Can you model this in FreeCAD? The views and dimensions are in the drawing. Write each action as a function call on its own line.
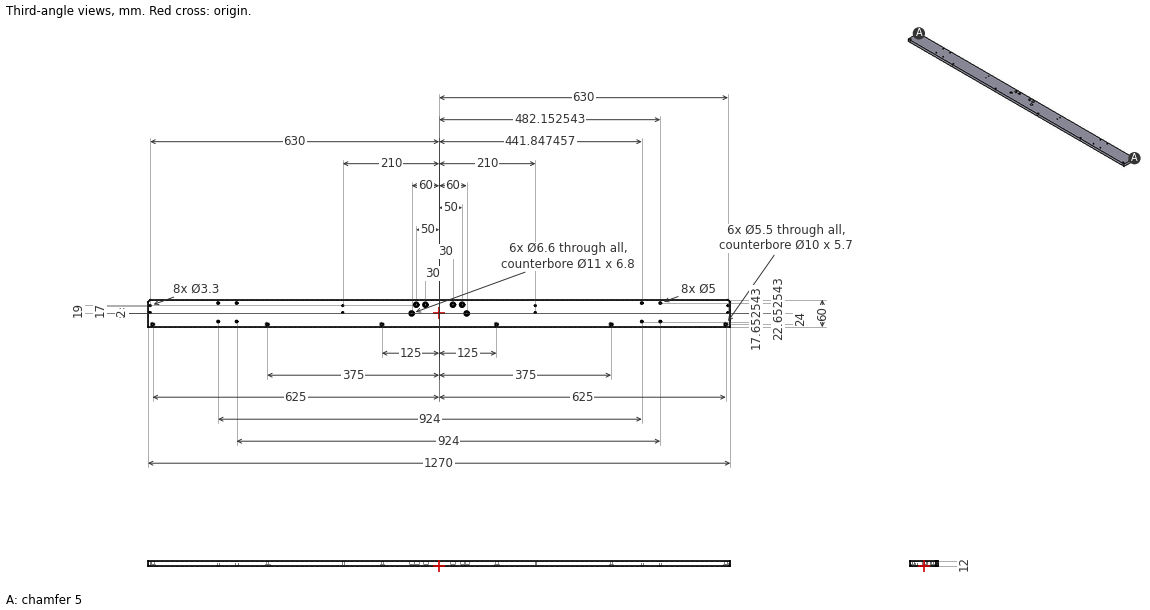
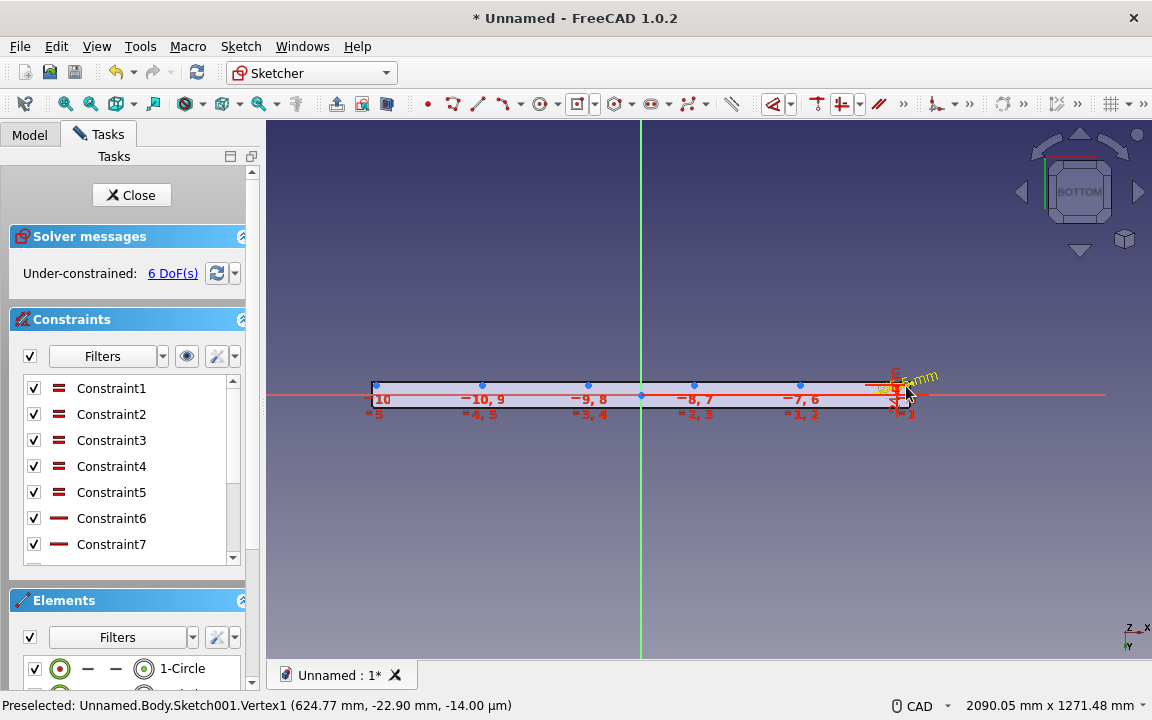
click(906, 385)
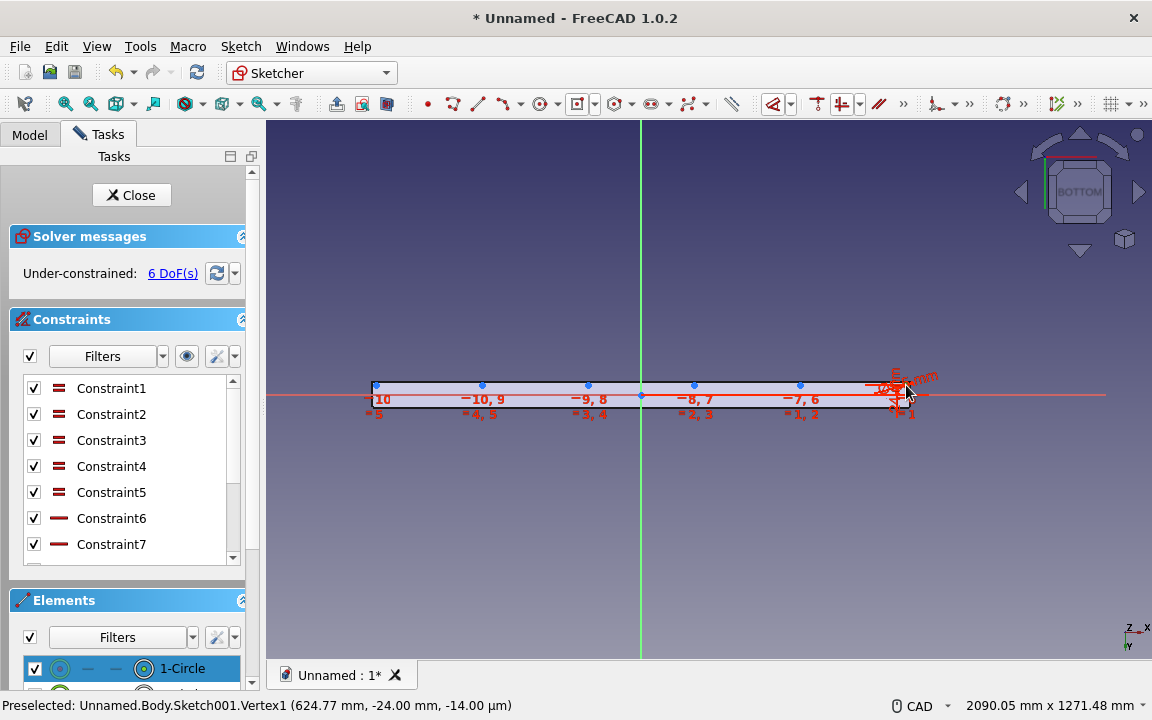
key(l)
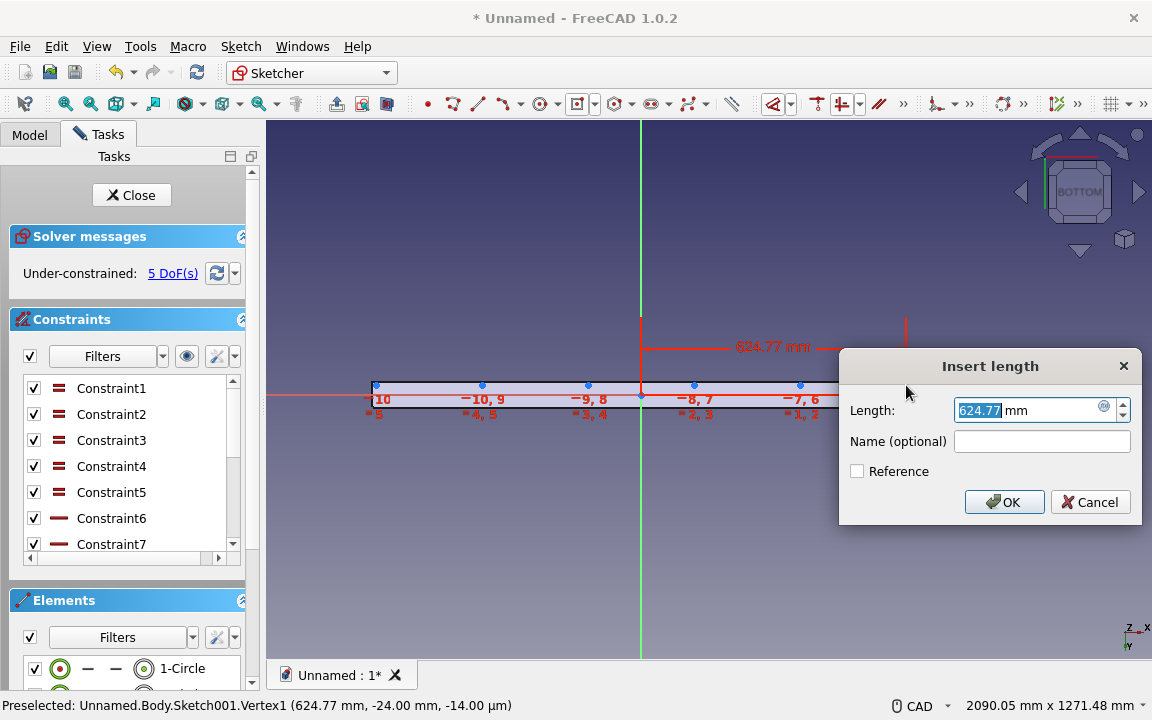
text(625)
key(Return)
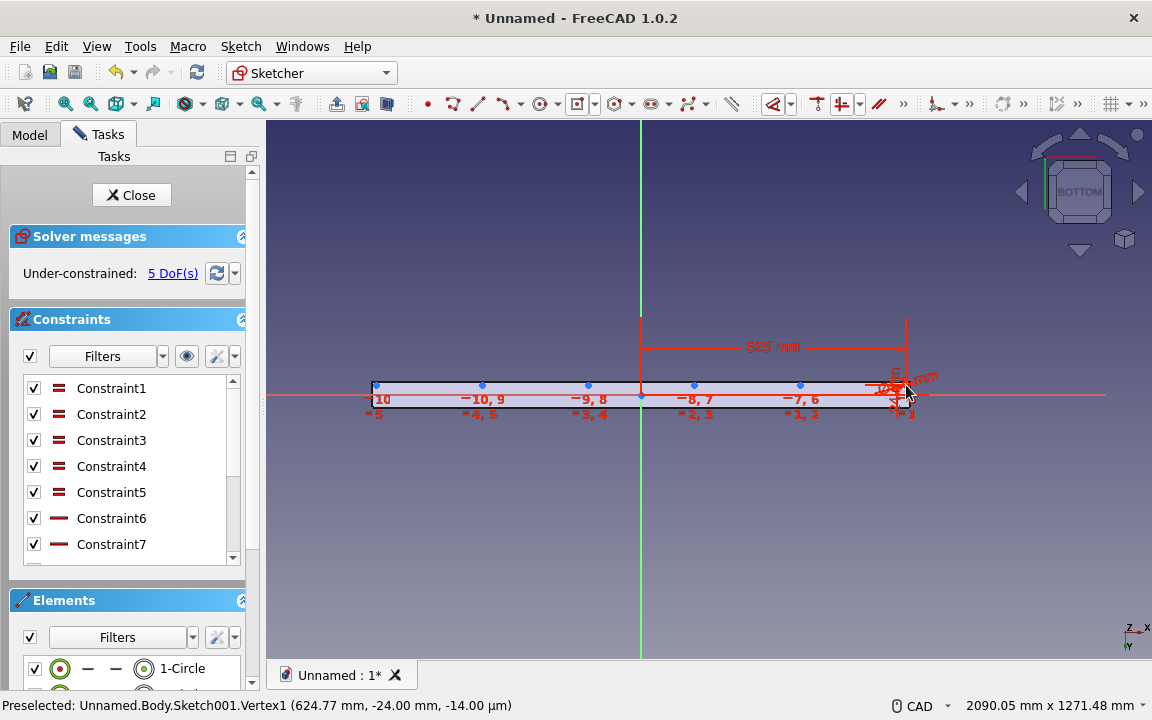
click(800, 385)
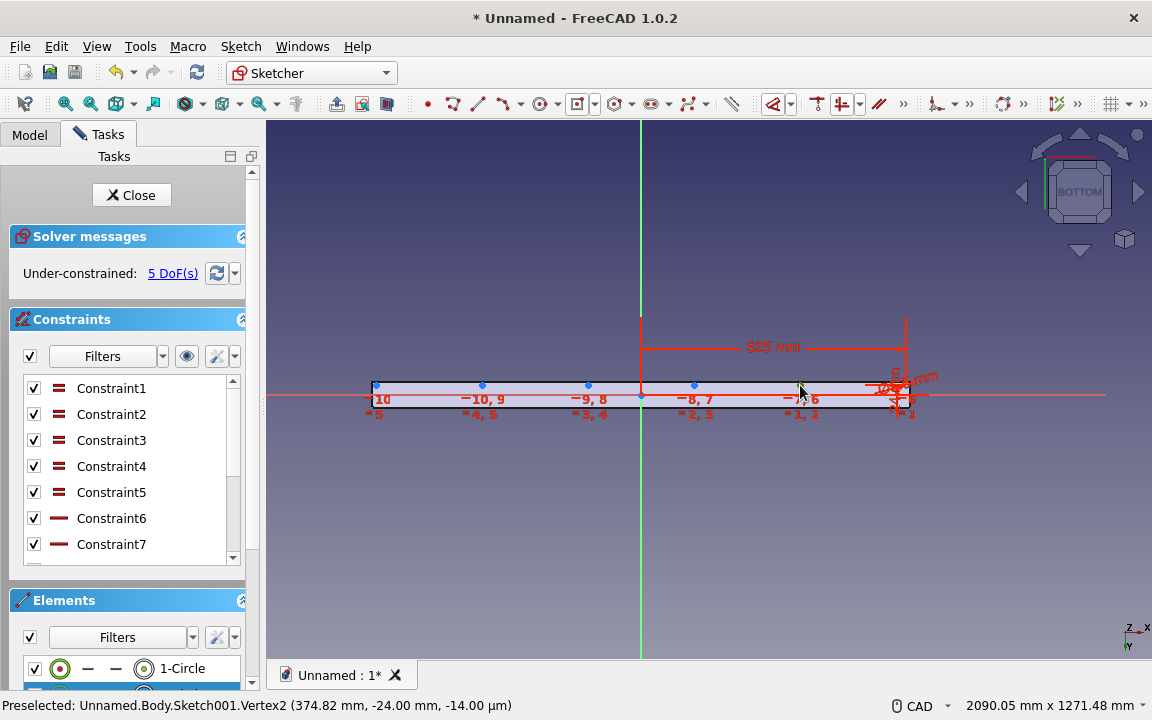
click(790, 104)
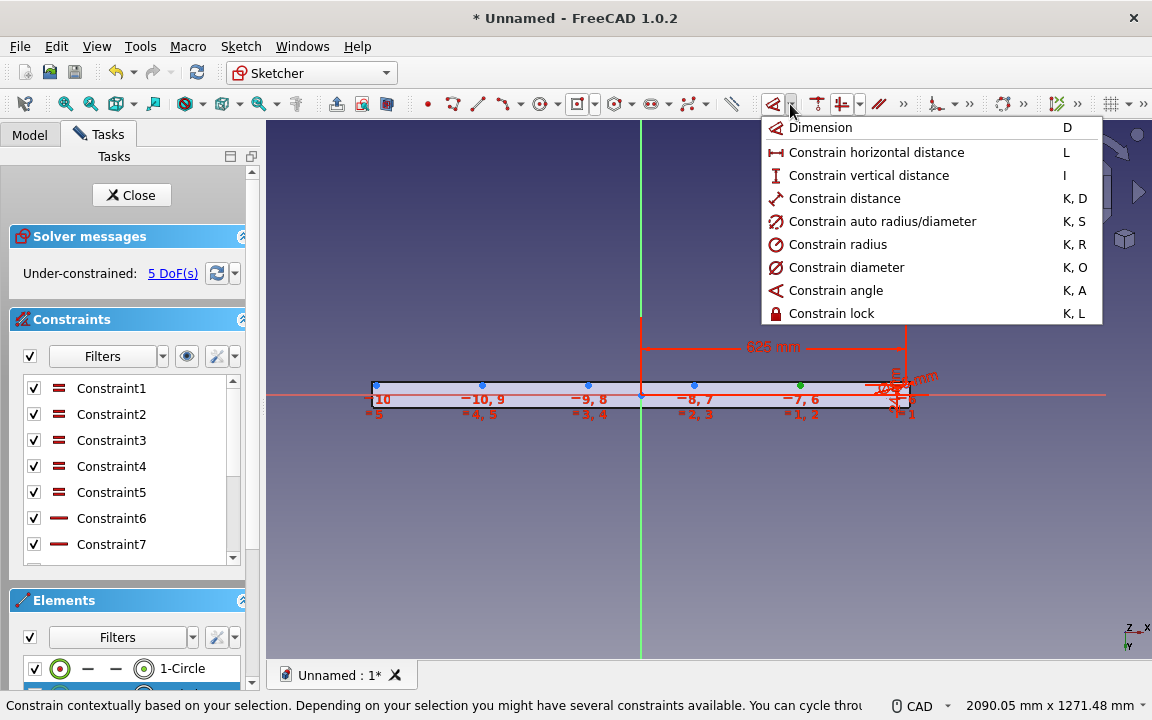
click(932, 152)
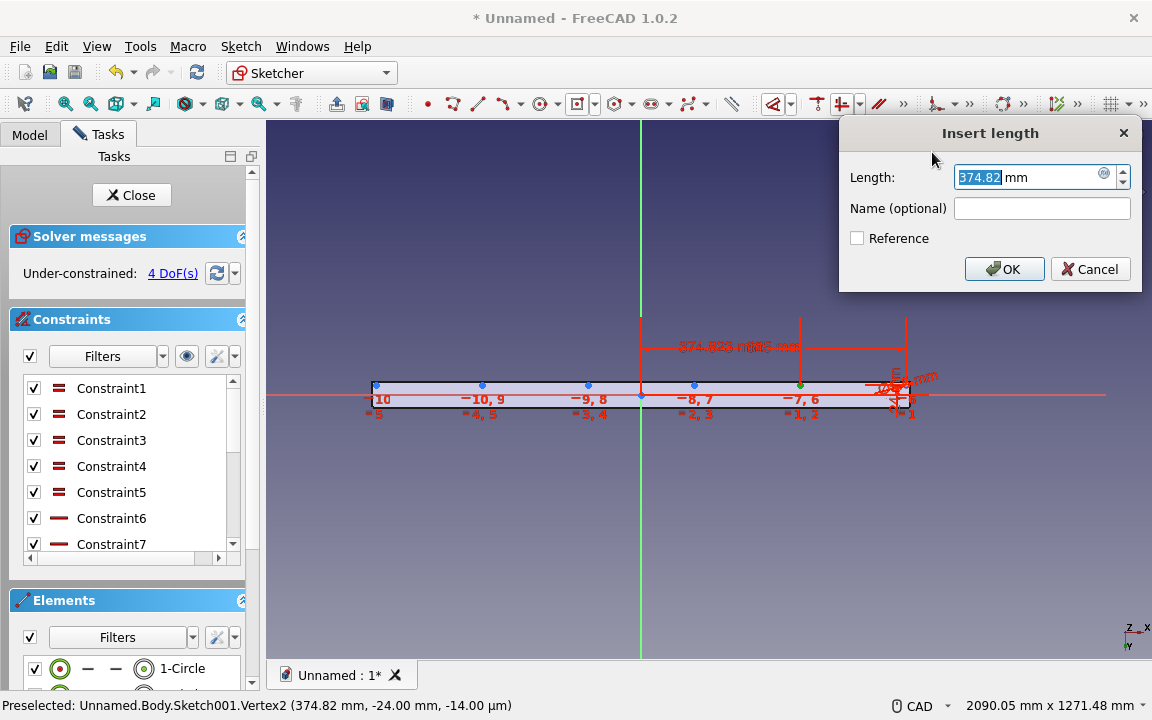
text(375)
key(Return)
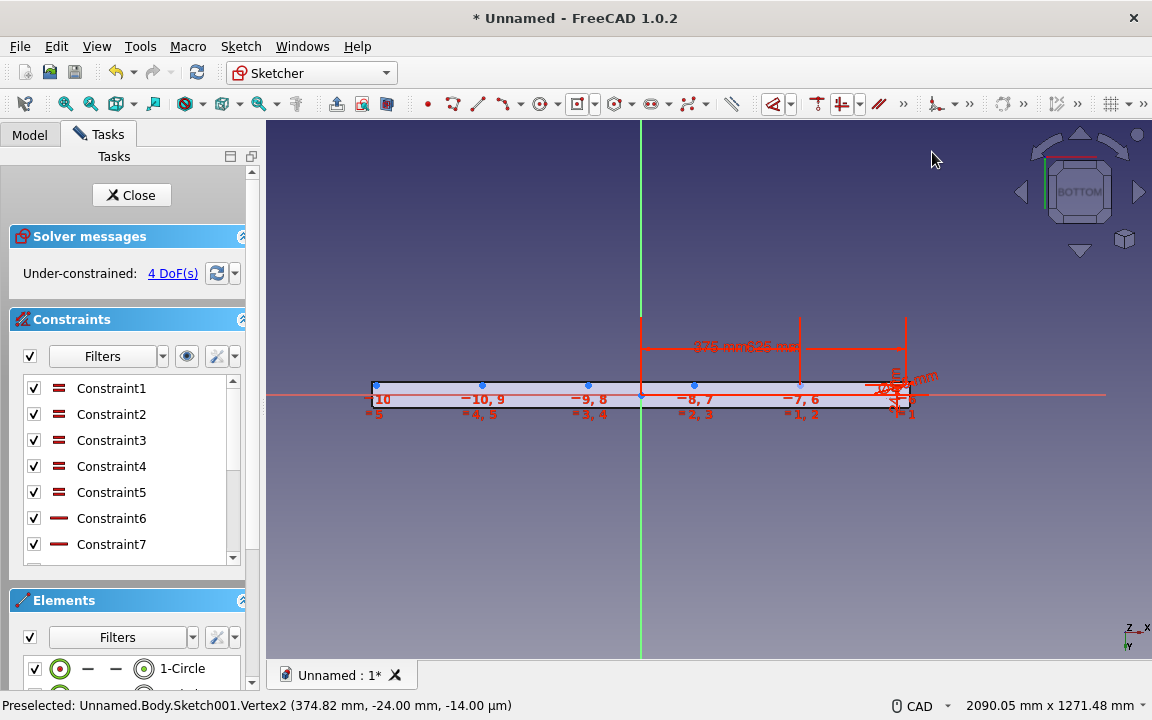
click(694, 385)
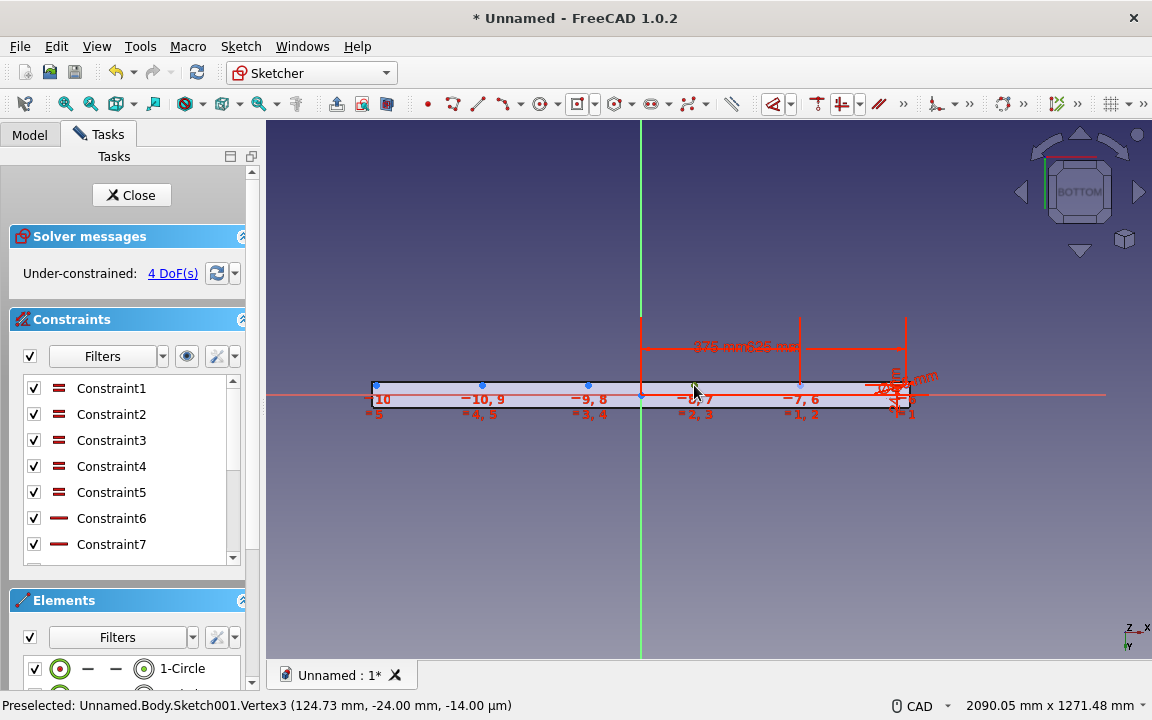
key(l)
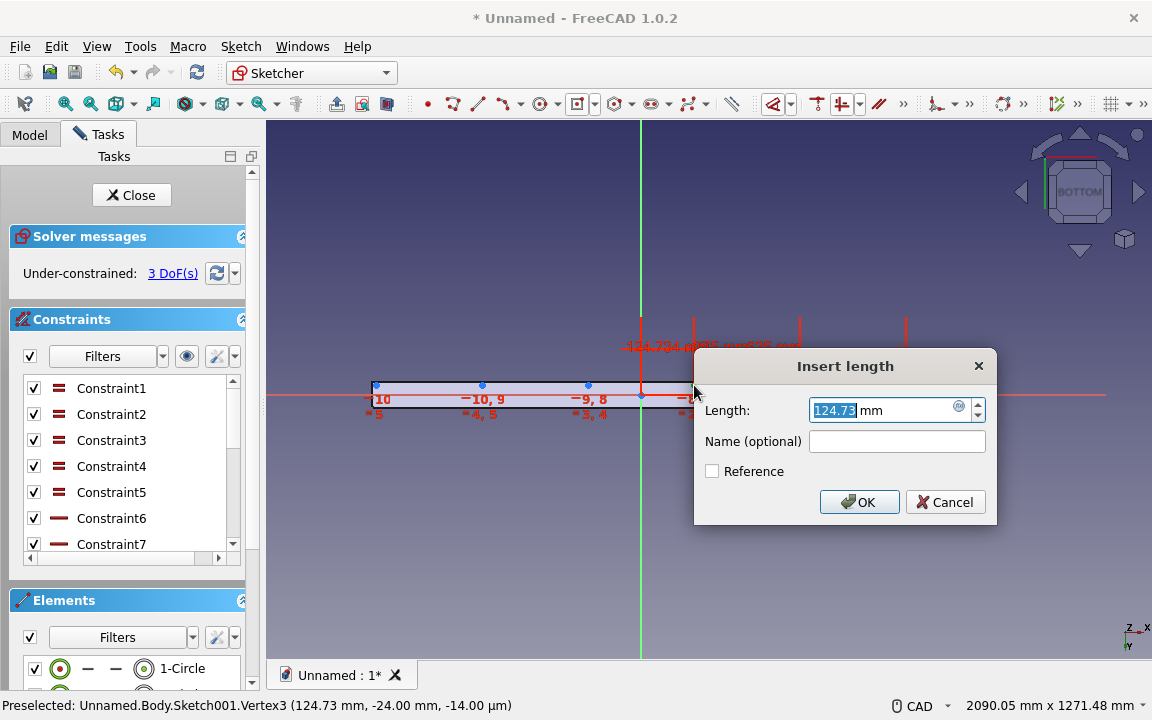
text(125)
key(Return)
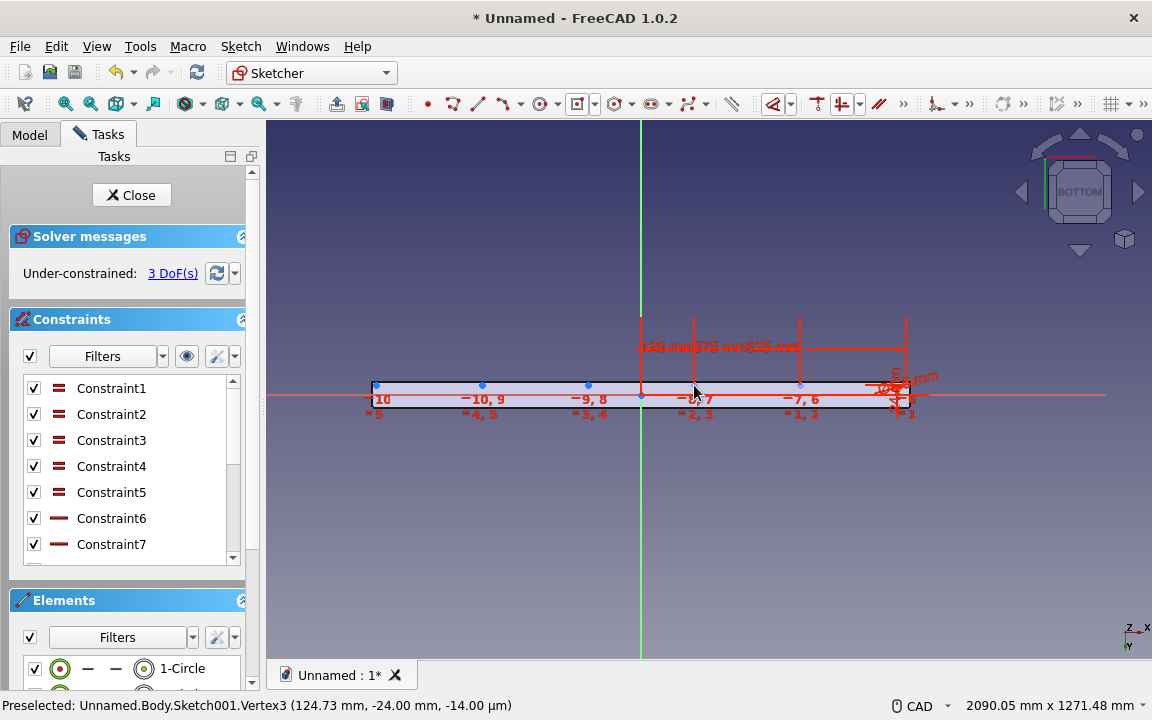
click(588, 385)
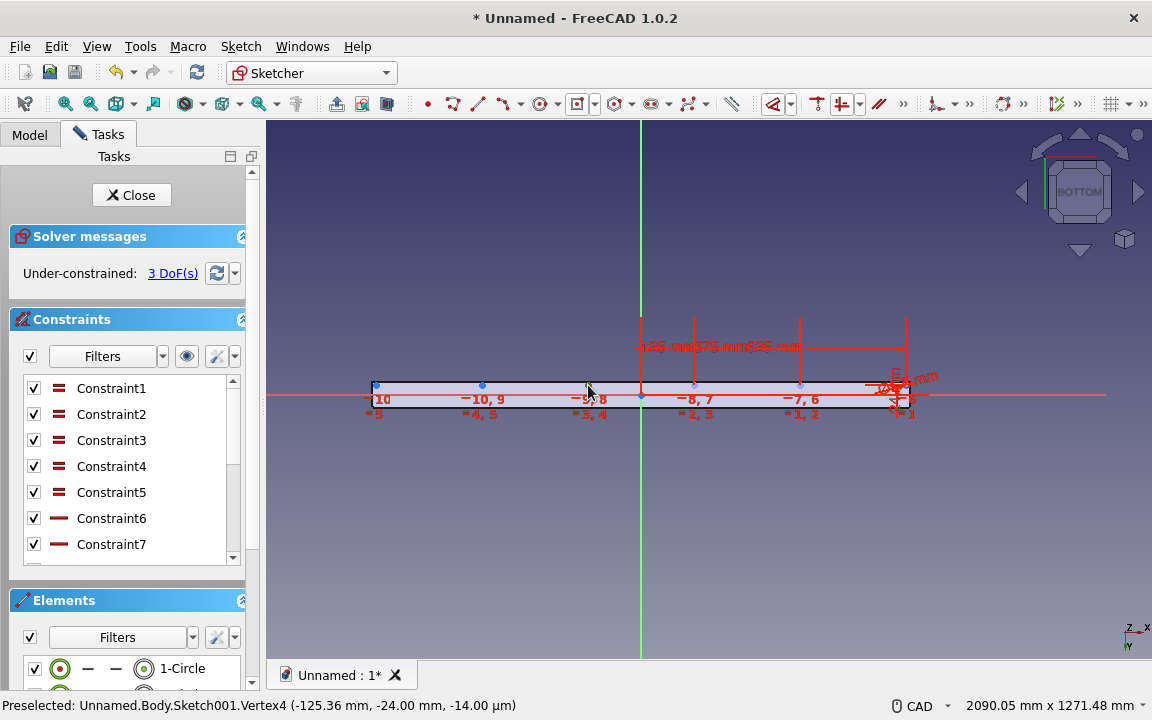
key(l)